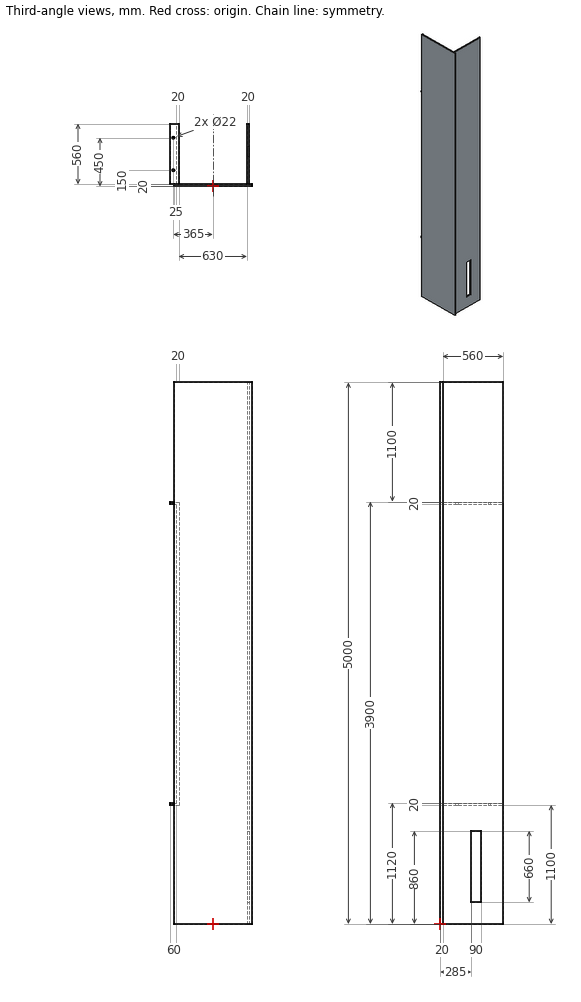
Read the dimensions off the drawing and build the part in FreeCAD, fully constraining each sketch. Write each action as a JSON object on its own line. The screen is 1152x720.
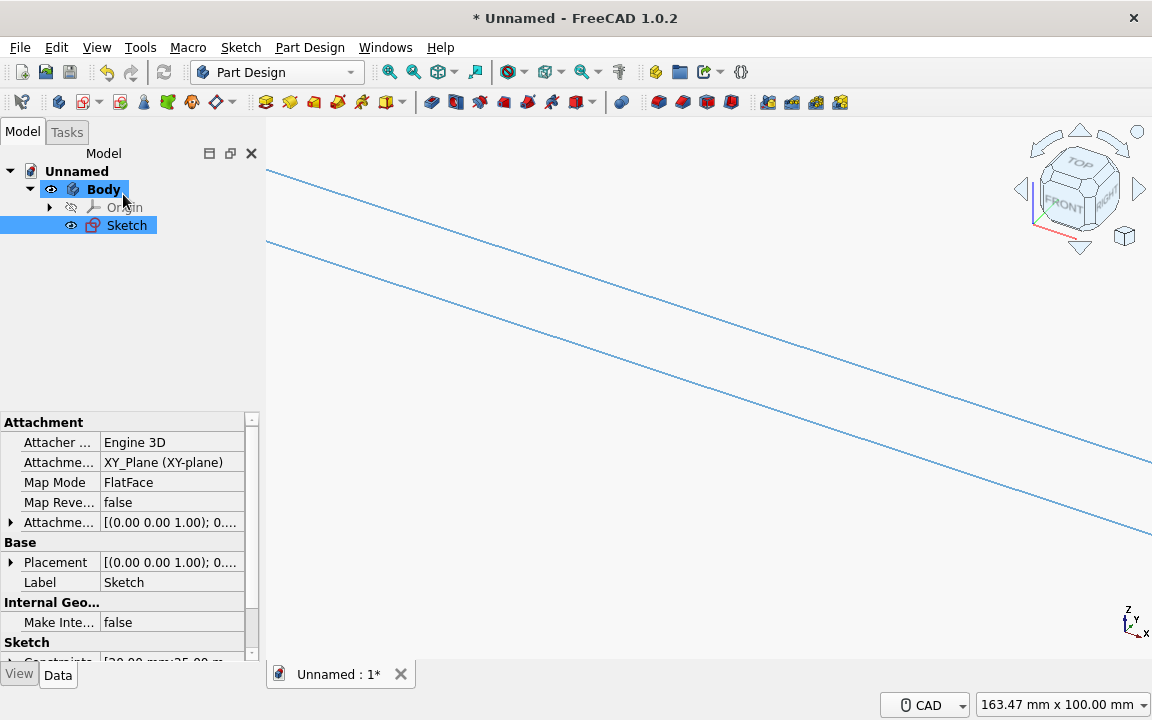
{"action": "left_click", "coordinate": [266, 102]}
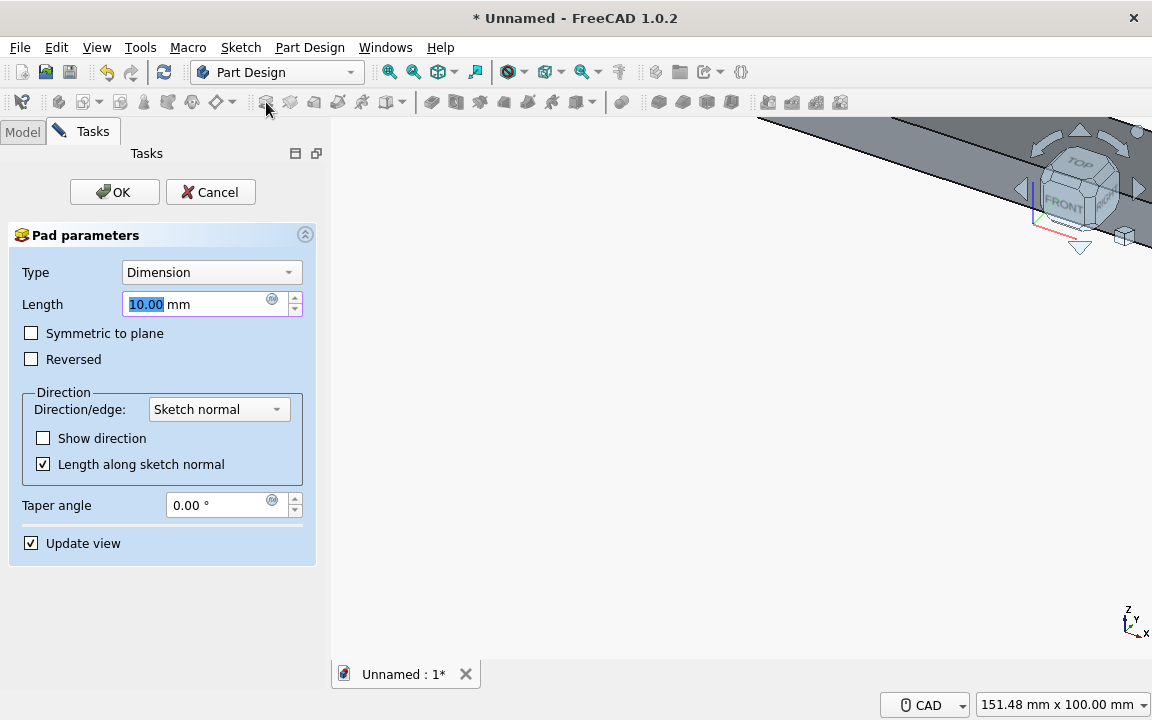
{"action": "type", "text": "5000"}
{"action": "key", "text": "Tab"}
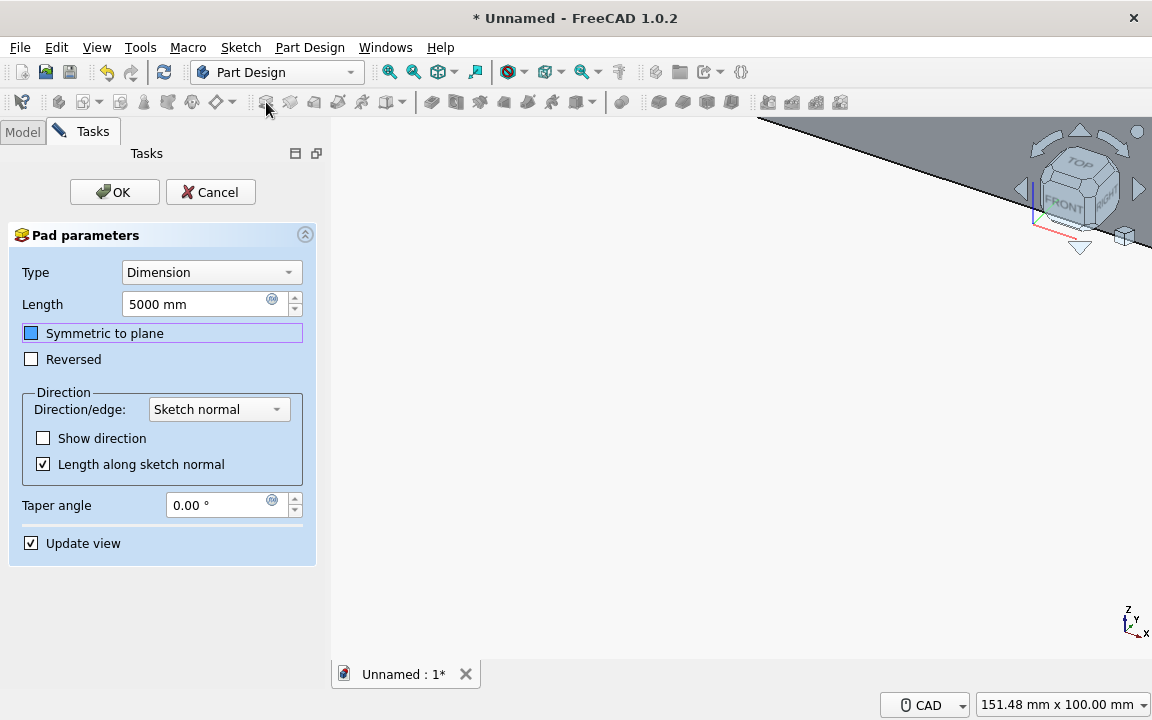
{"action": "left_click", "coordinate": [115, 192]}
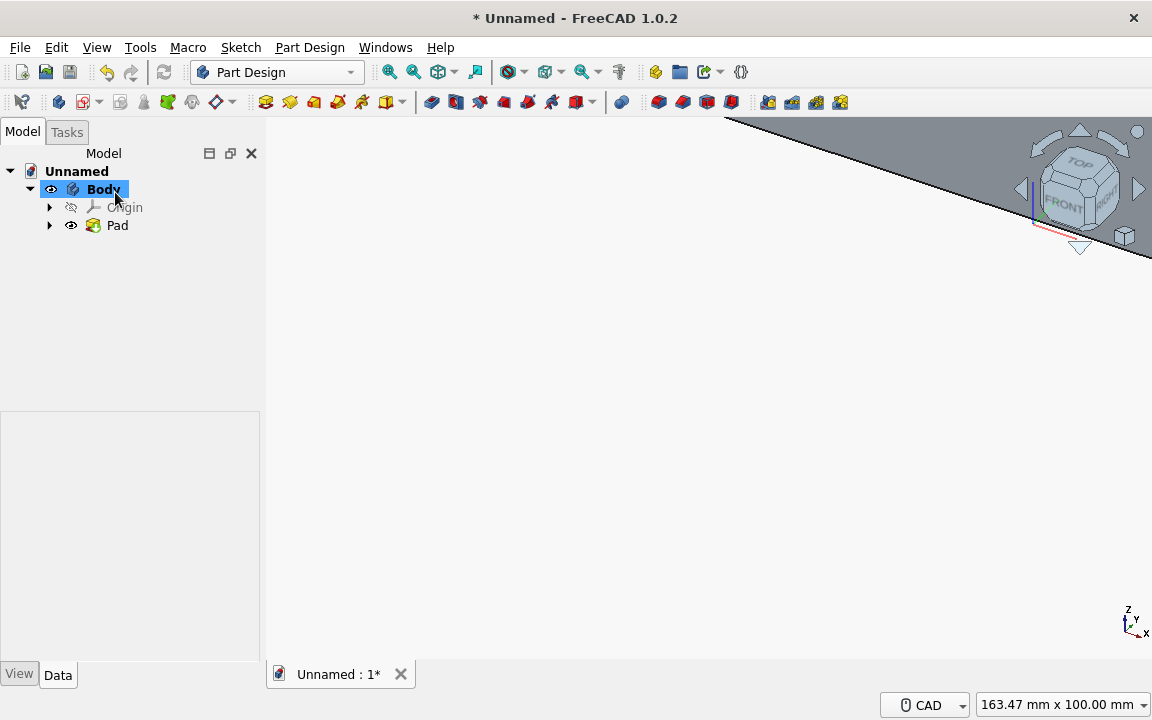
{"action": "left_click", "coordinate": [390, 72]}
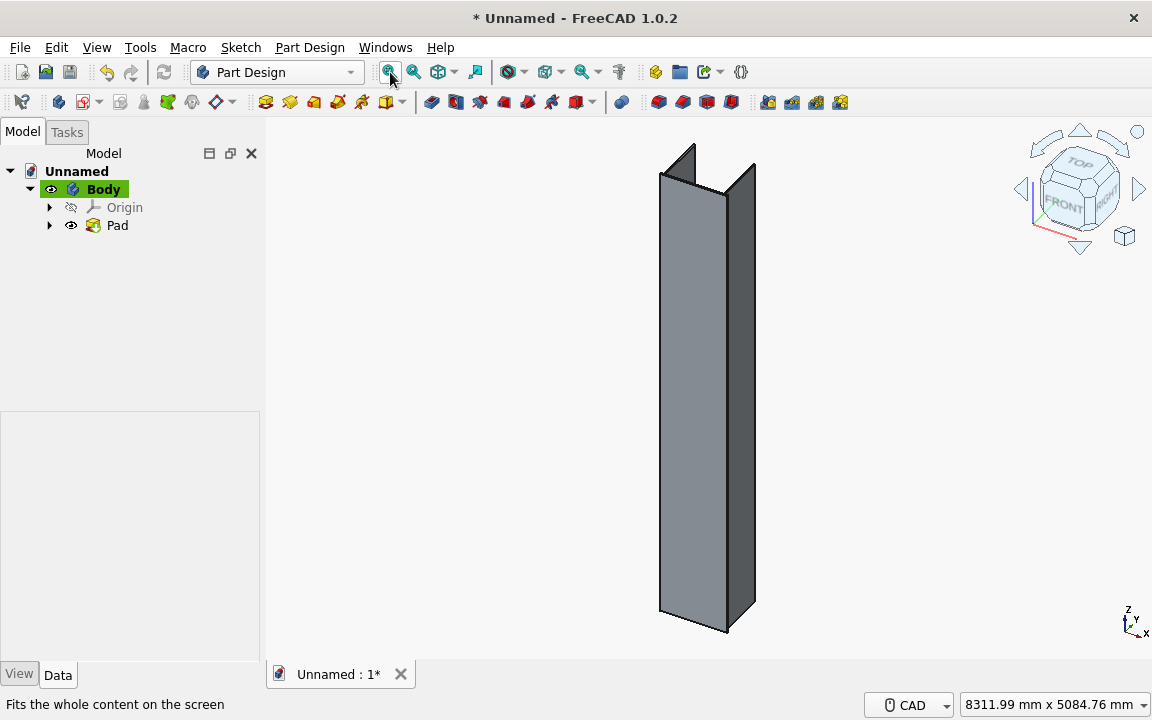
{"action": "left_click", "coordinate": [740, 210]}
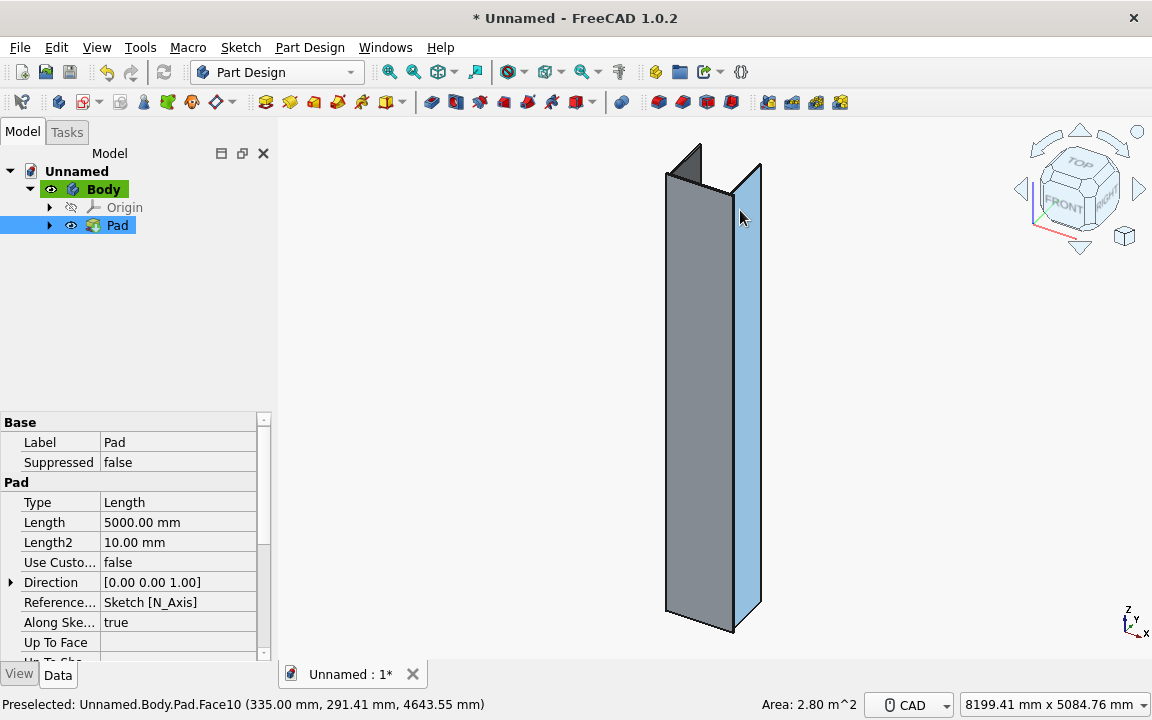
{"action": "left_click", "coordinate": [84, 102]}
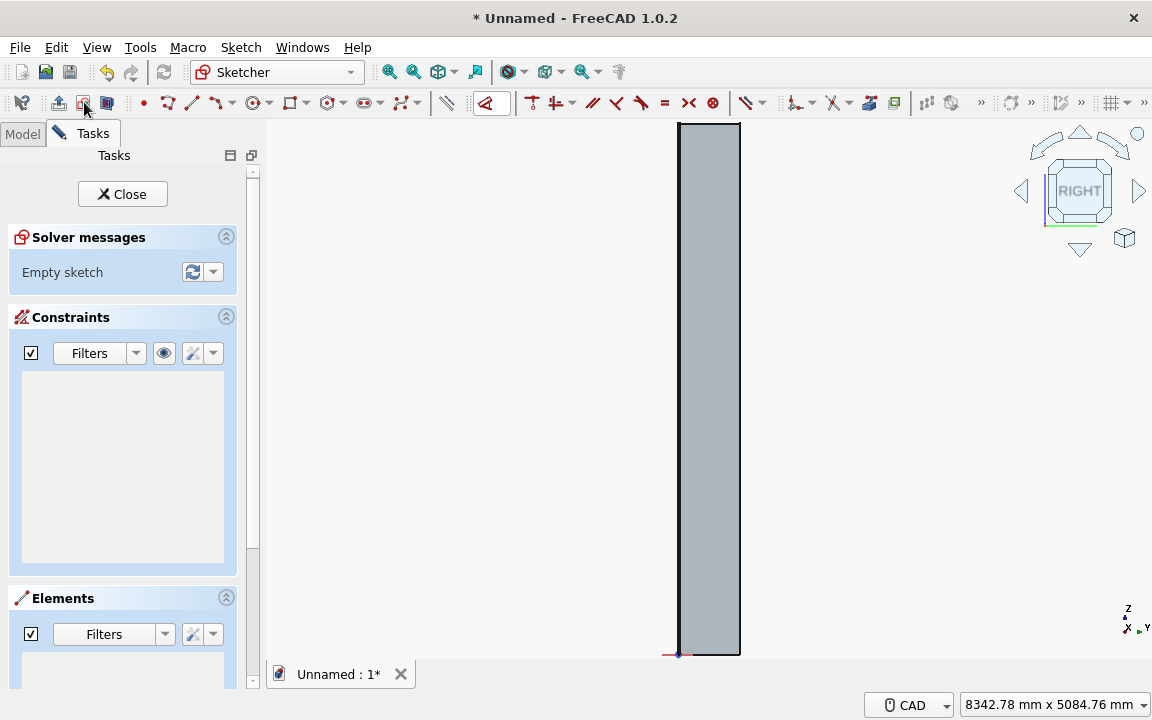
{"action": "left_click", "coordinate": [108, 104]}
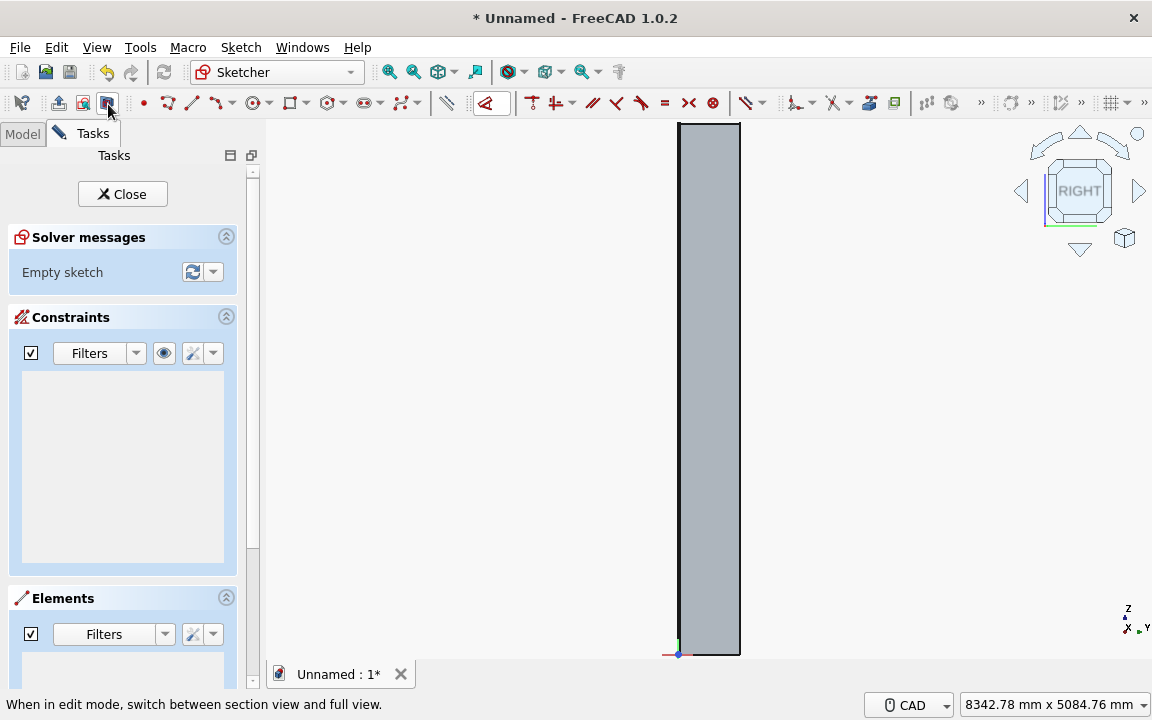
{"action": "scroll", "coordinate": [640, 389], "scroll_direction": "down", "scroll_amount": 5}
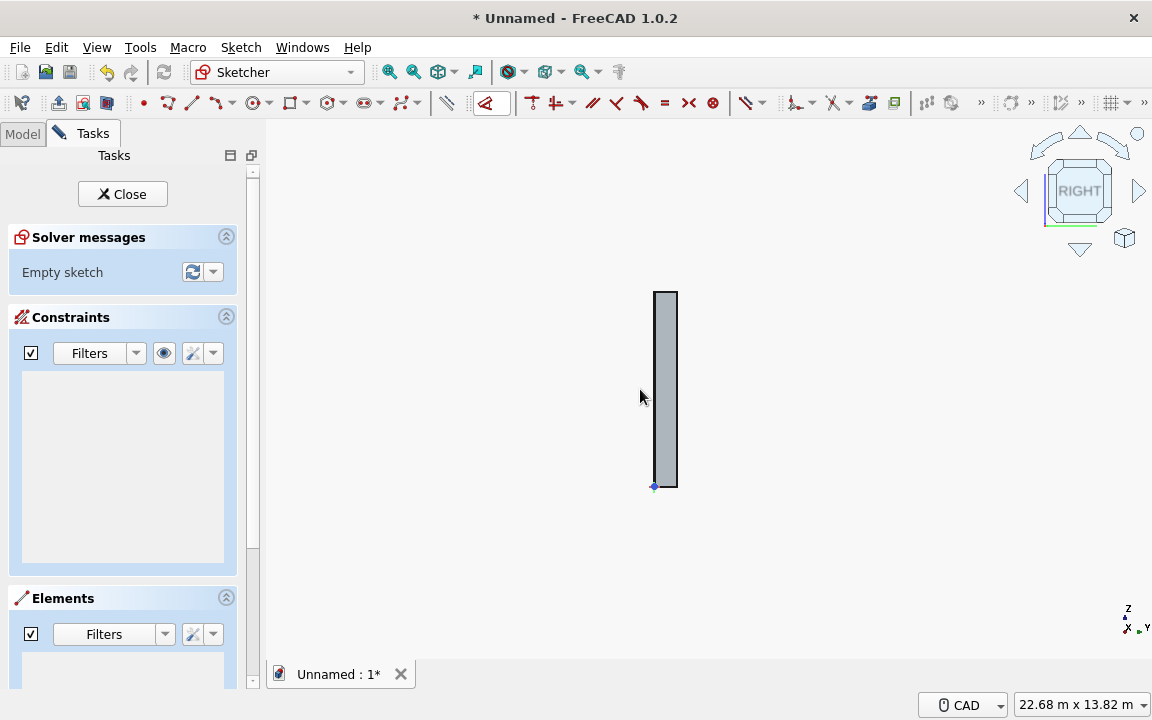
{"action": "scroll", "coordinate": [664, 478], "scroll_direction": "up", "scroll_amount": 12}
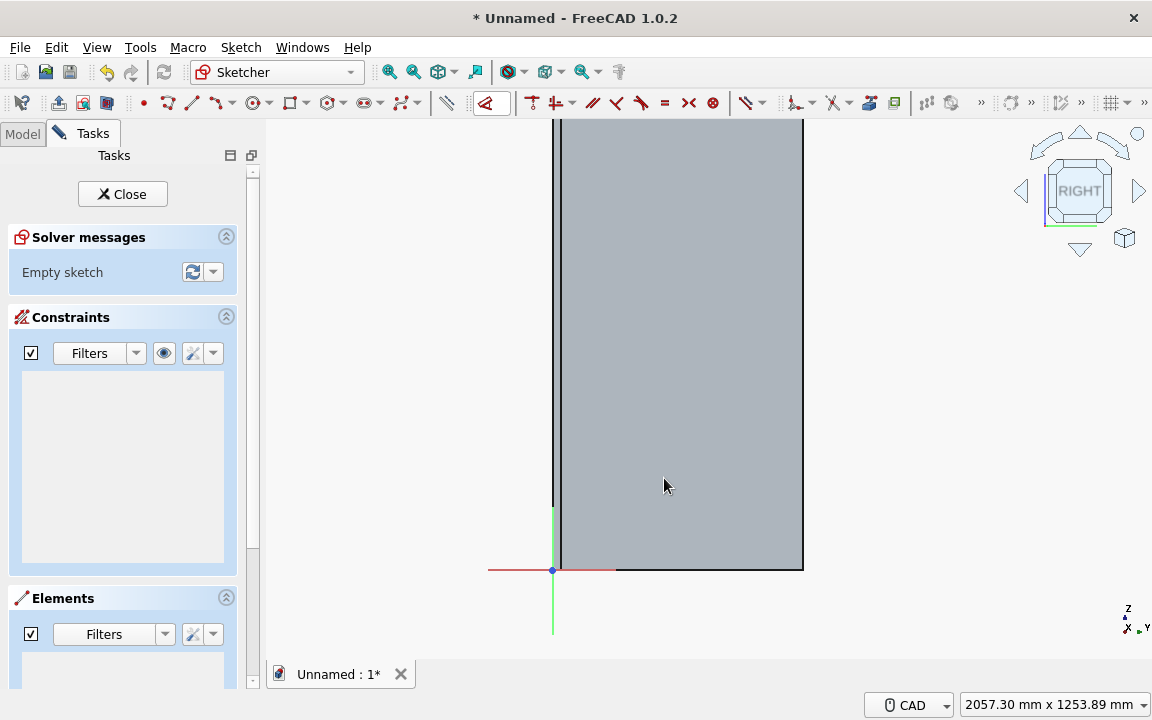
{"action": "left_click", "coordinate": [290, 104]}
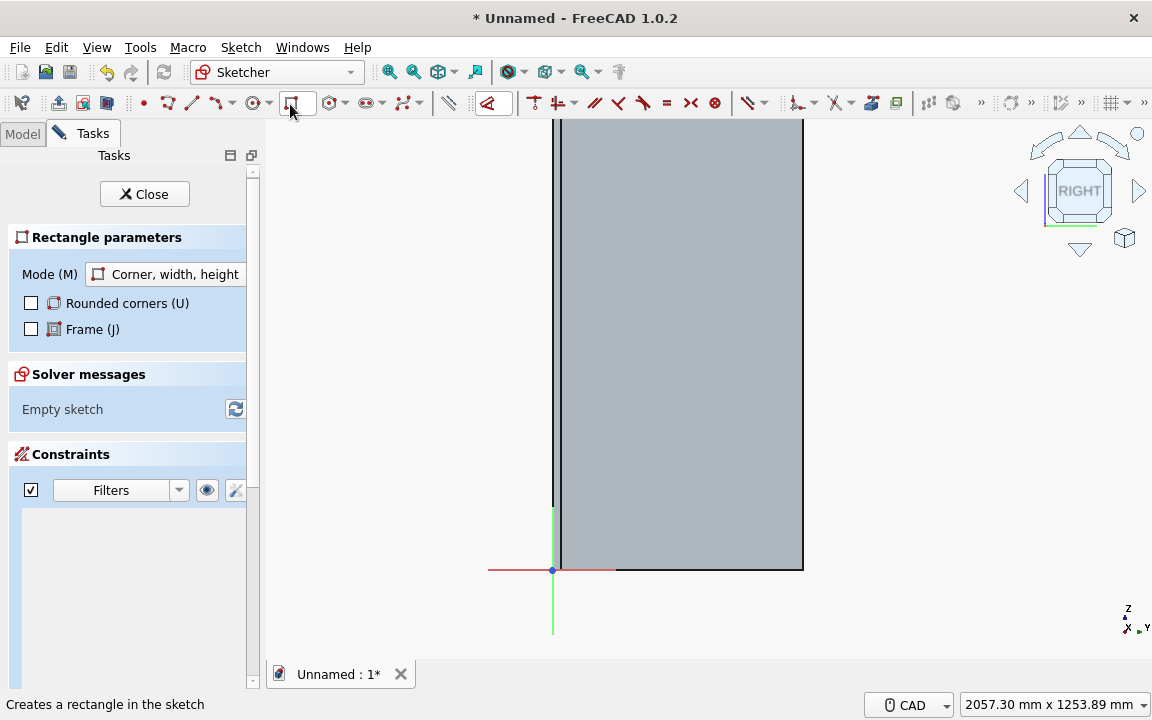
{"action": "left_click", "coordinate": [676, 200]}
{"action": "mouse_move", "coordinate": [714, 484]}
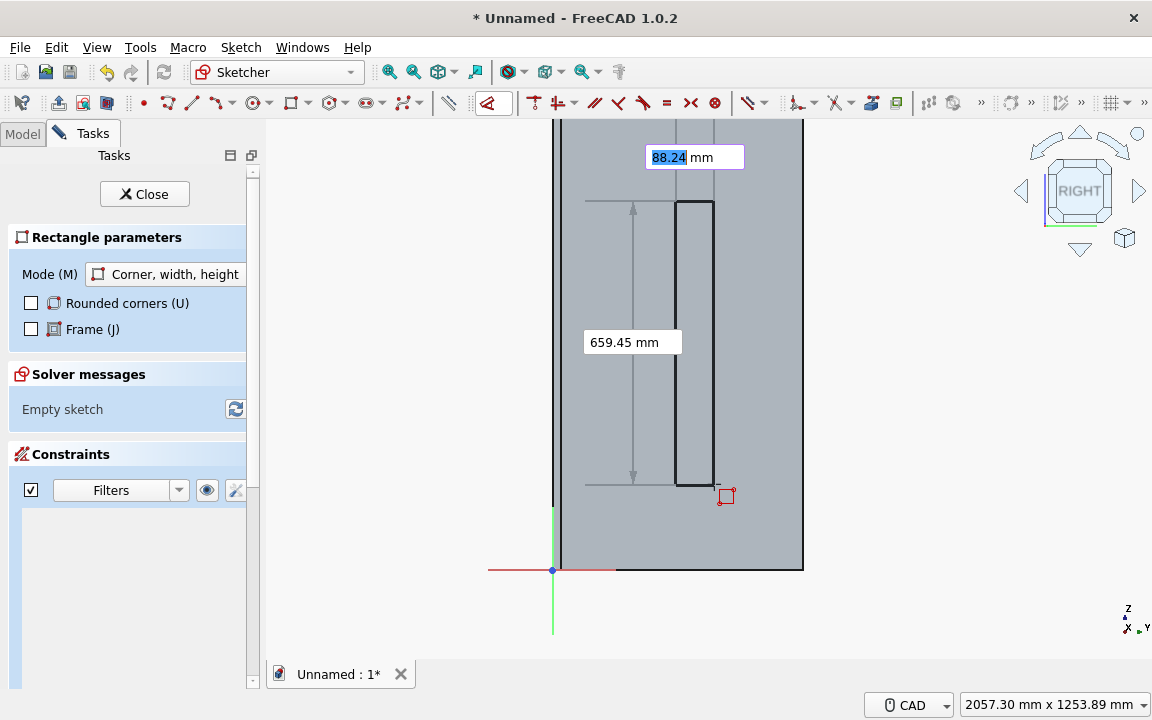
{"action": "type", "text": "90"}
{"action": "key", "text": "Tab"}
{"action": "type", "text": "660"}
{"action": "key", "text": "Return"}
{"action": "key", "text": "Escape"}